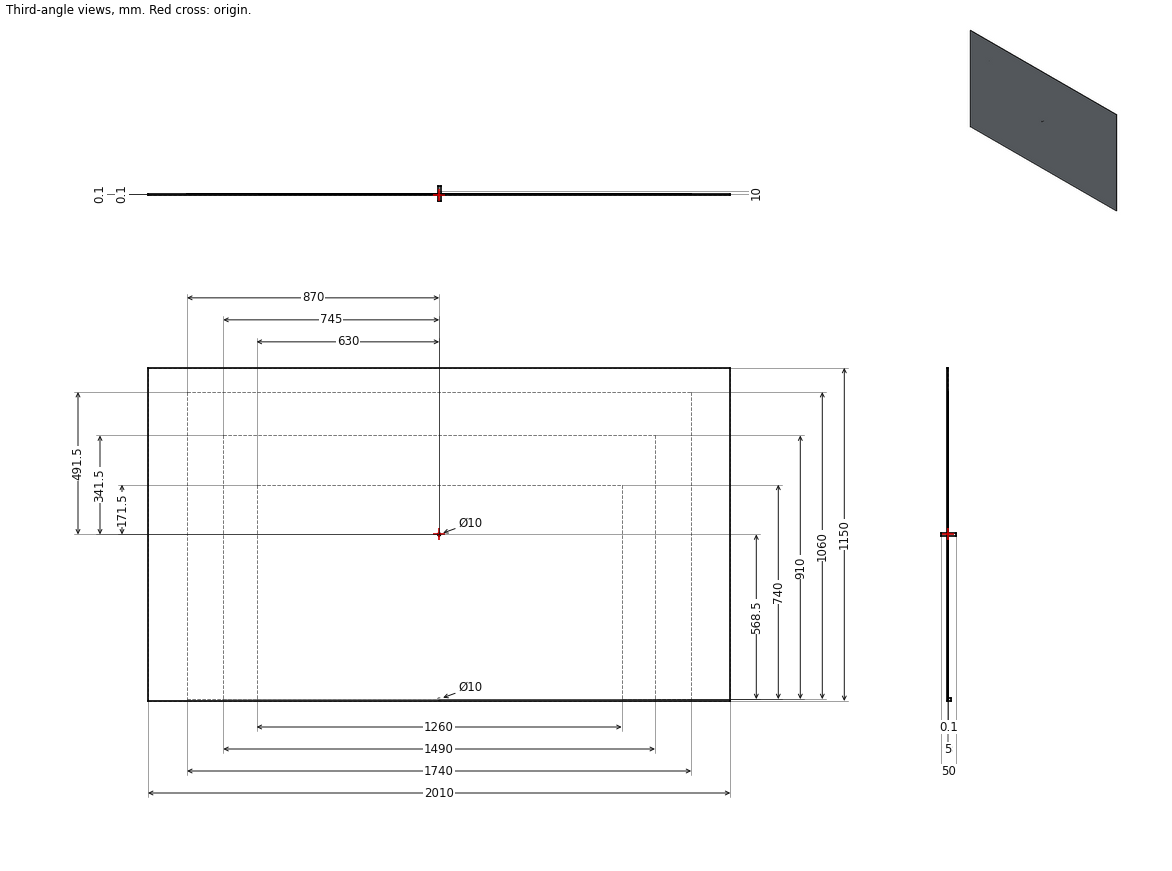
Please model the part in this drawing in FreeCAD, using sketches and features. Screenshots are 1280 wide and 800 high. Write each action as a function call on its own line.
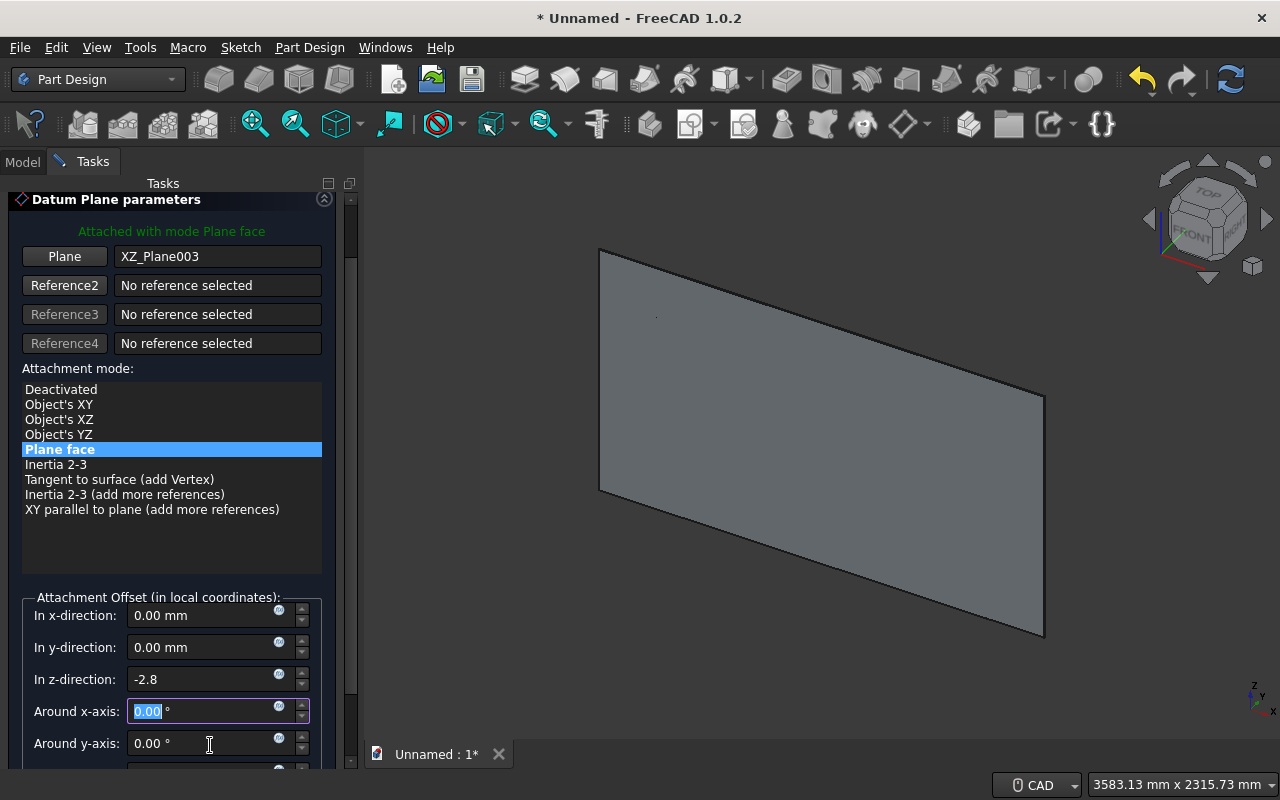
scroll(351, 480, up, 2)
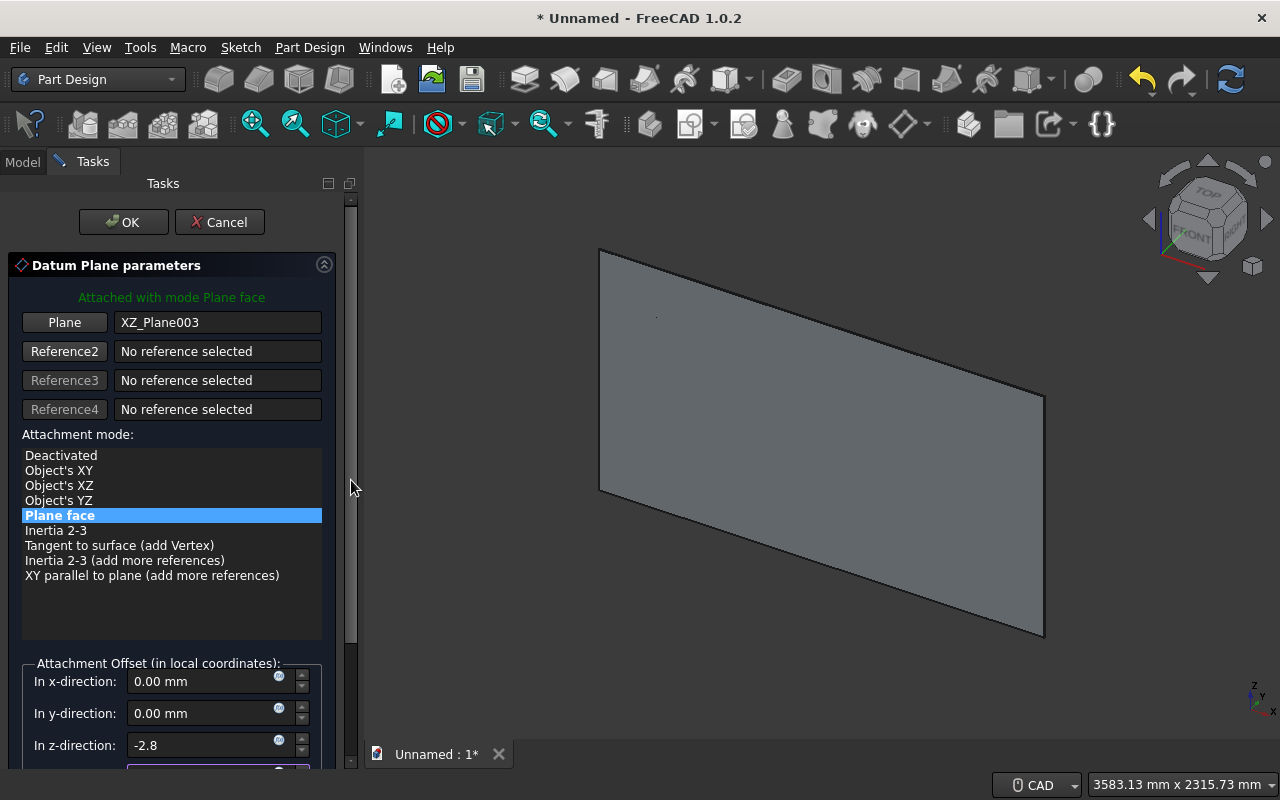
click(124, 222)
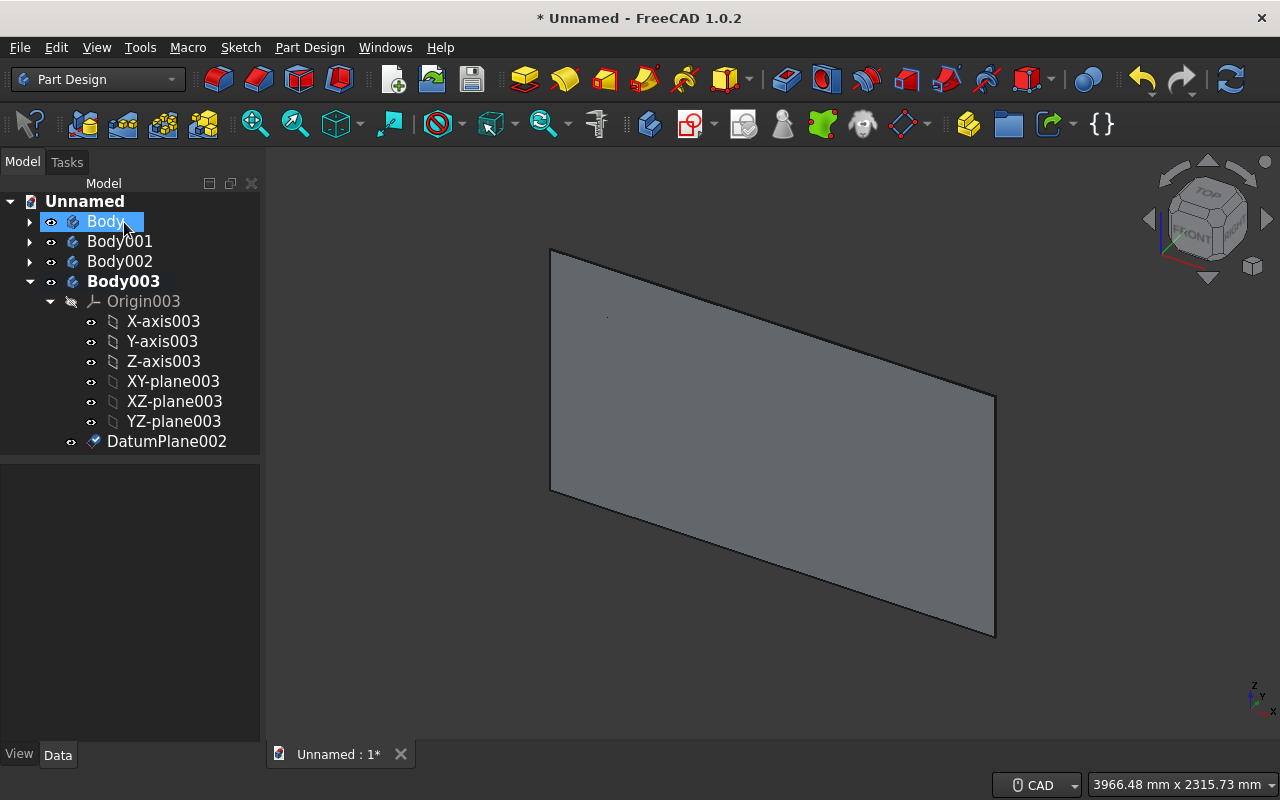
click(116, 442)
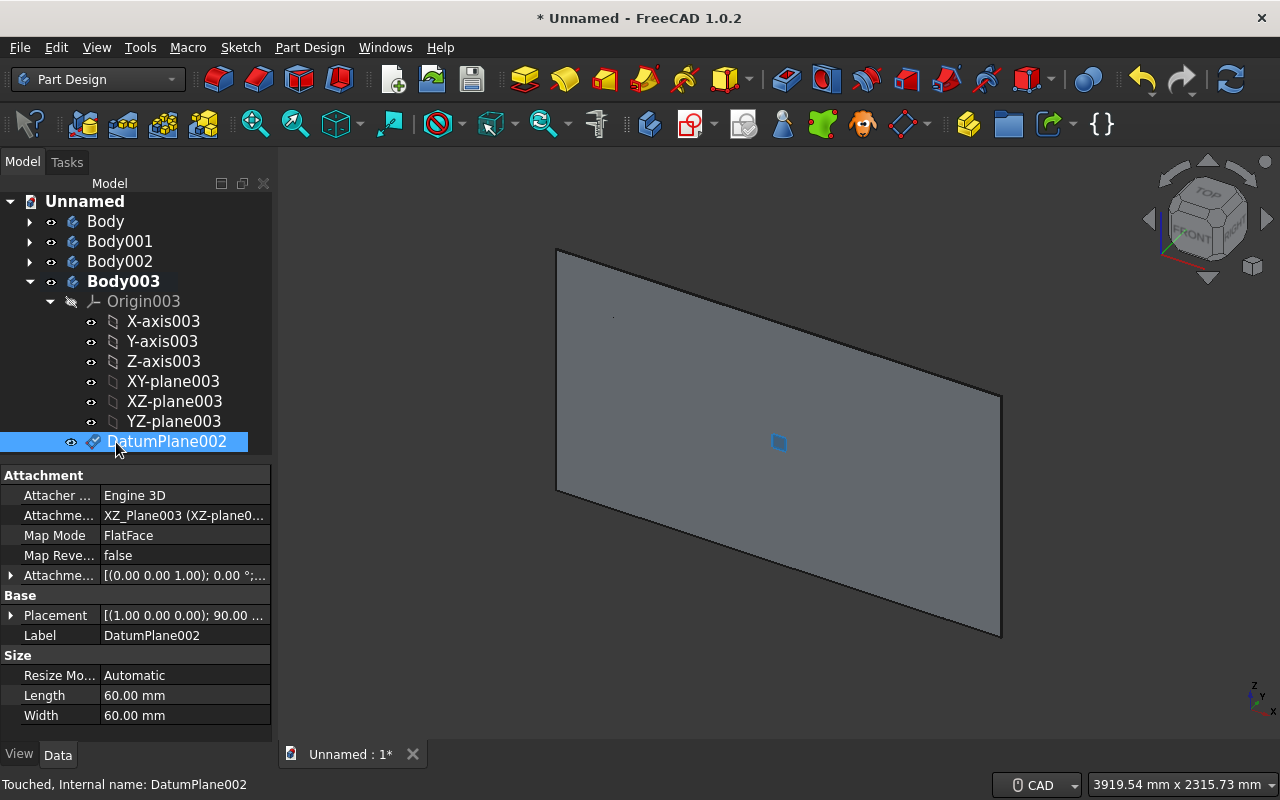
click(690, 124)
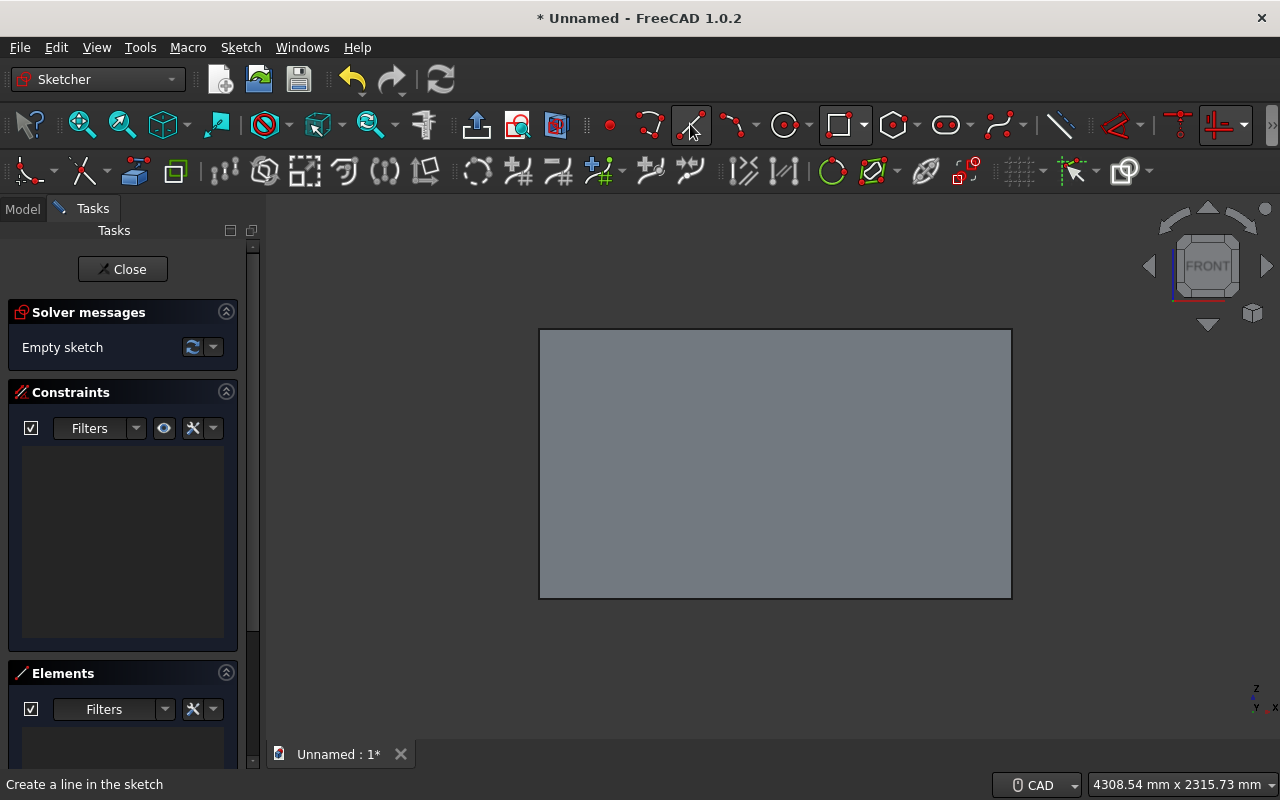
scroll(861, 564, up, 3)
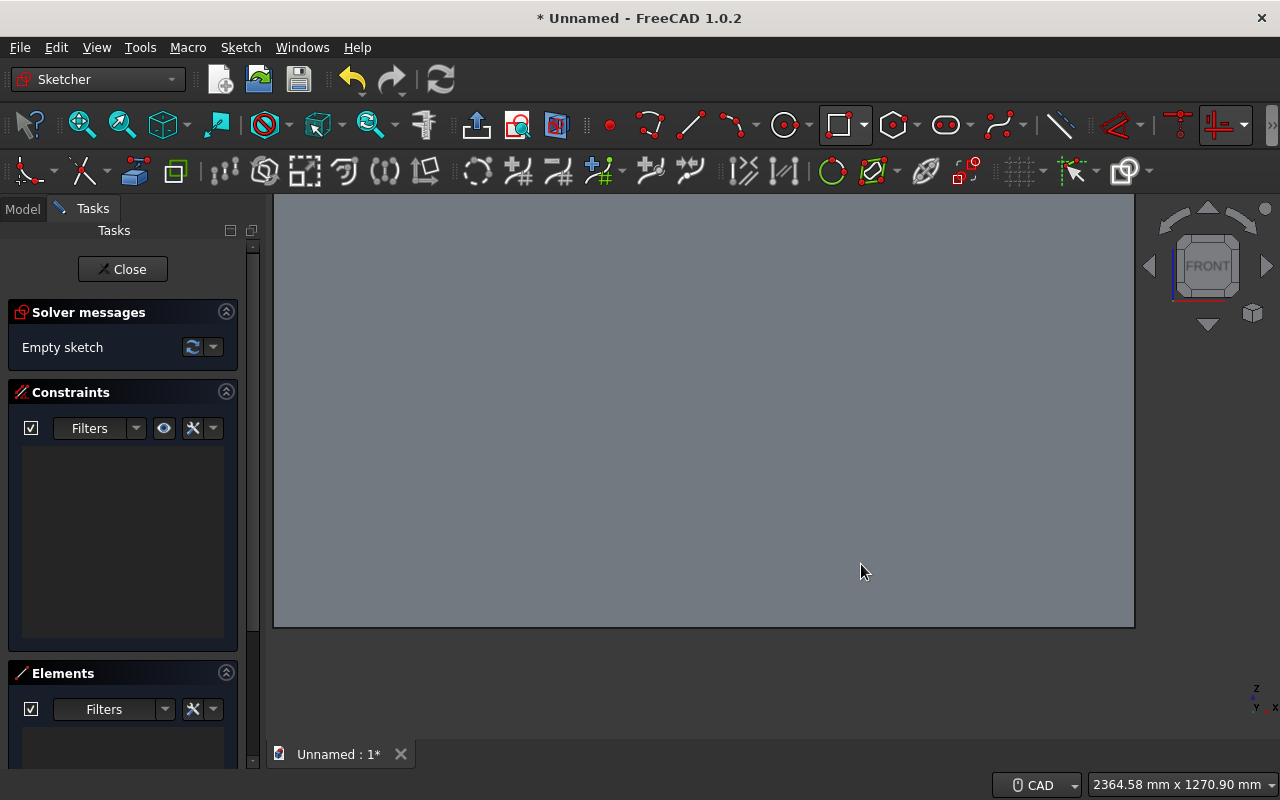
click(840, 126)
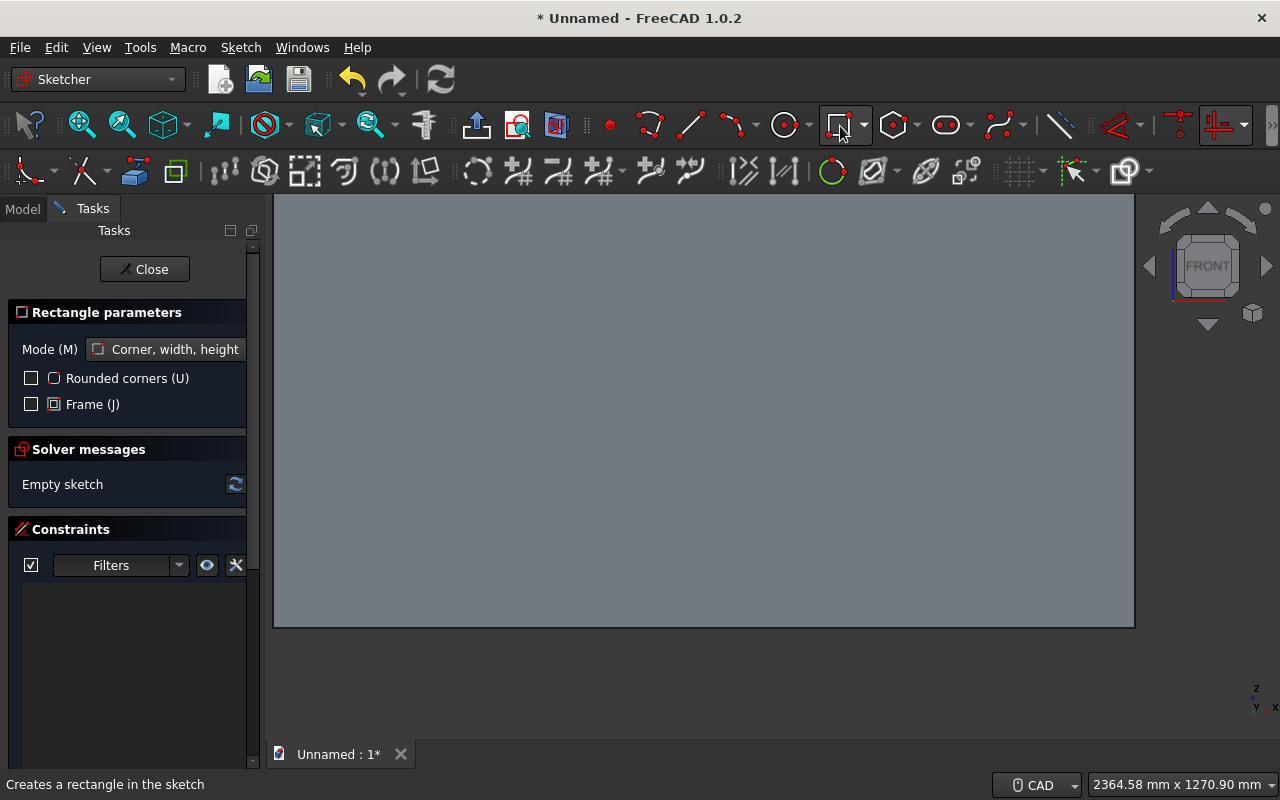
click(434, 307)
move(974, 625)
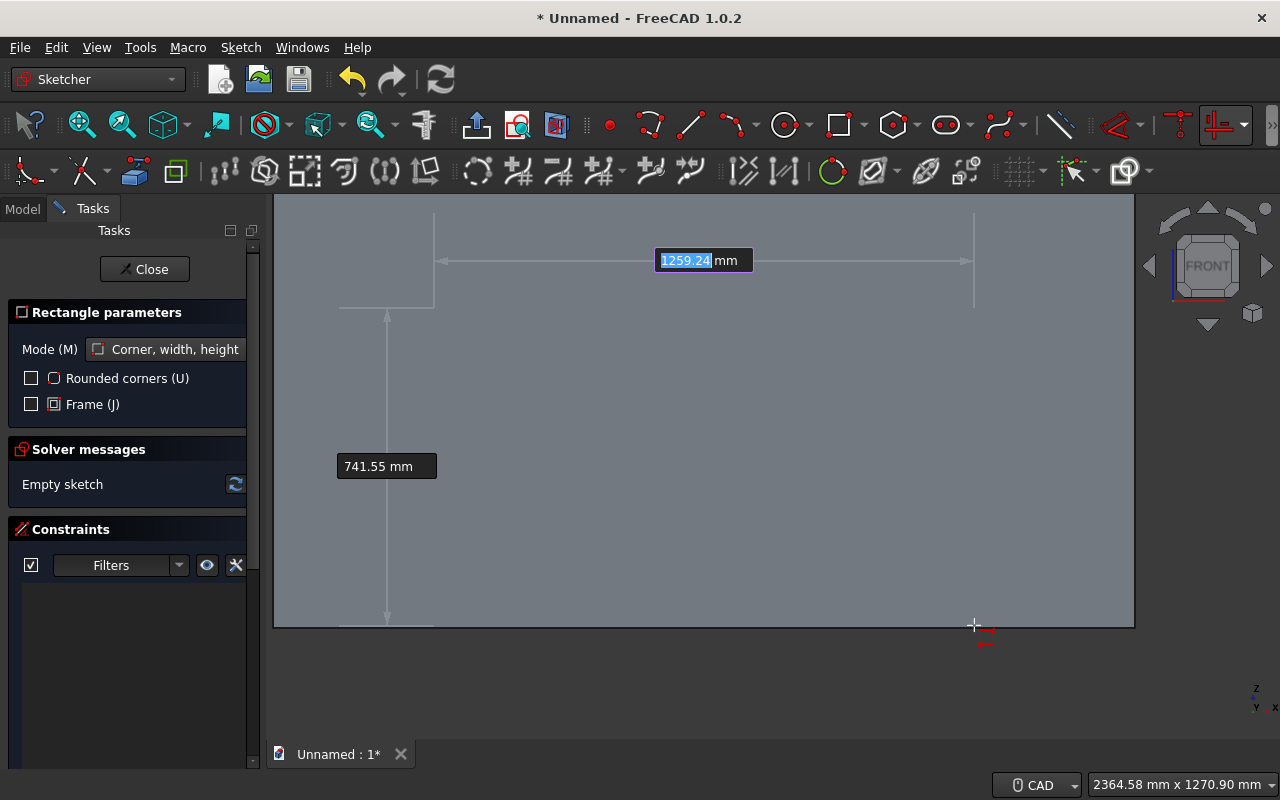
text(1260)
key(Tab)
text(740)
key(Return)
key(Escape)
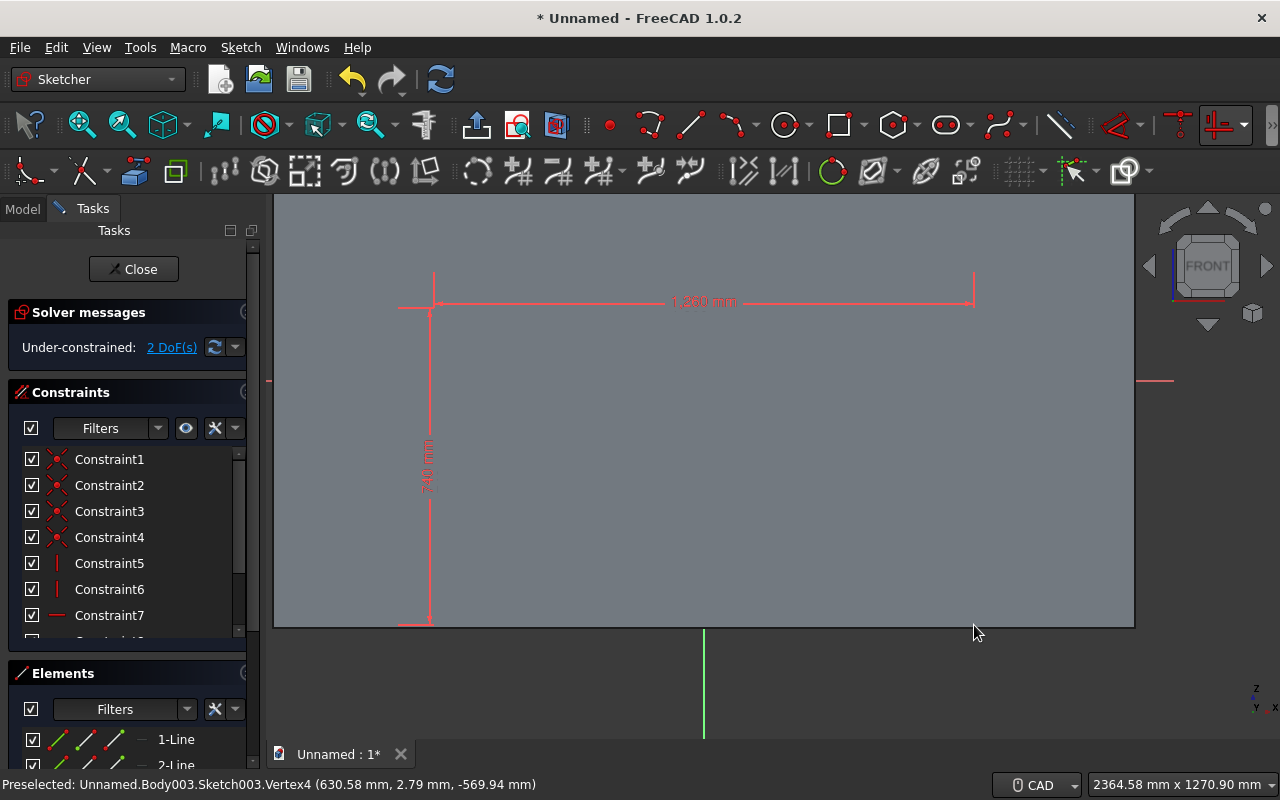
click(1116, 126)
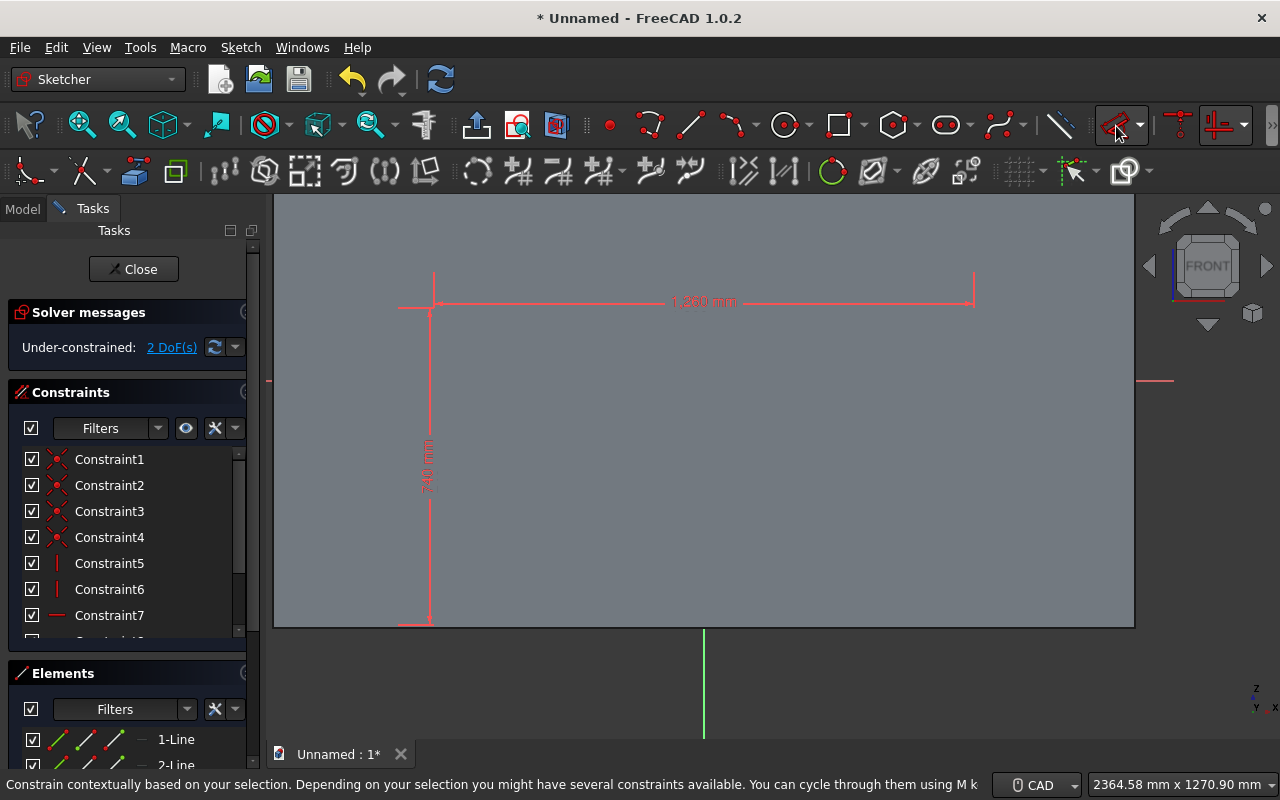
click(434, 308)
click(569, 274)